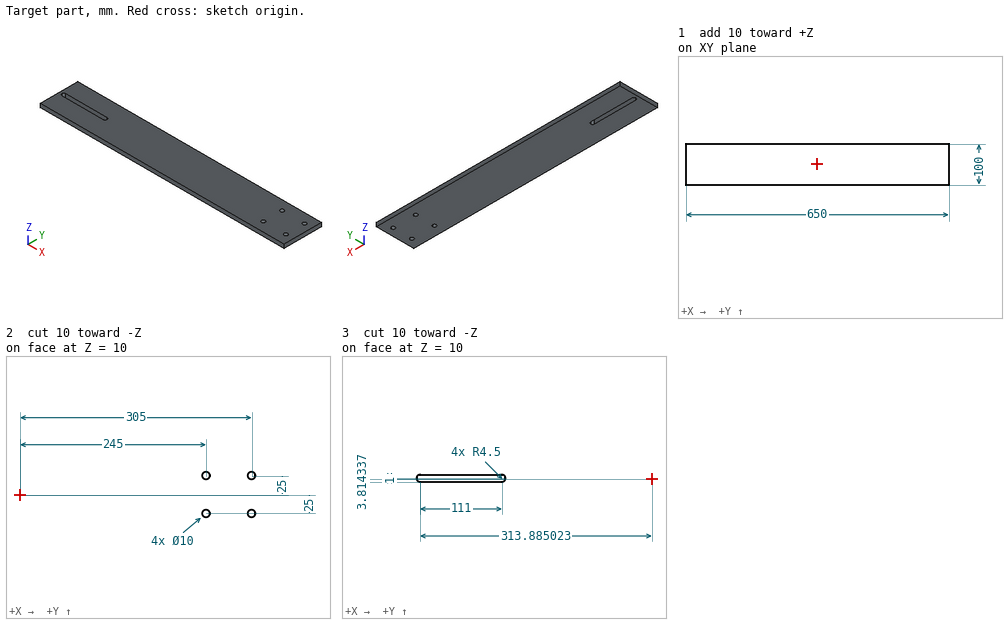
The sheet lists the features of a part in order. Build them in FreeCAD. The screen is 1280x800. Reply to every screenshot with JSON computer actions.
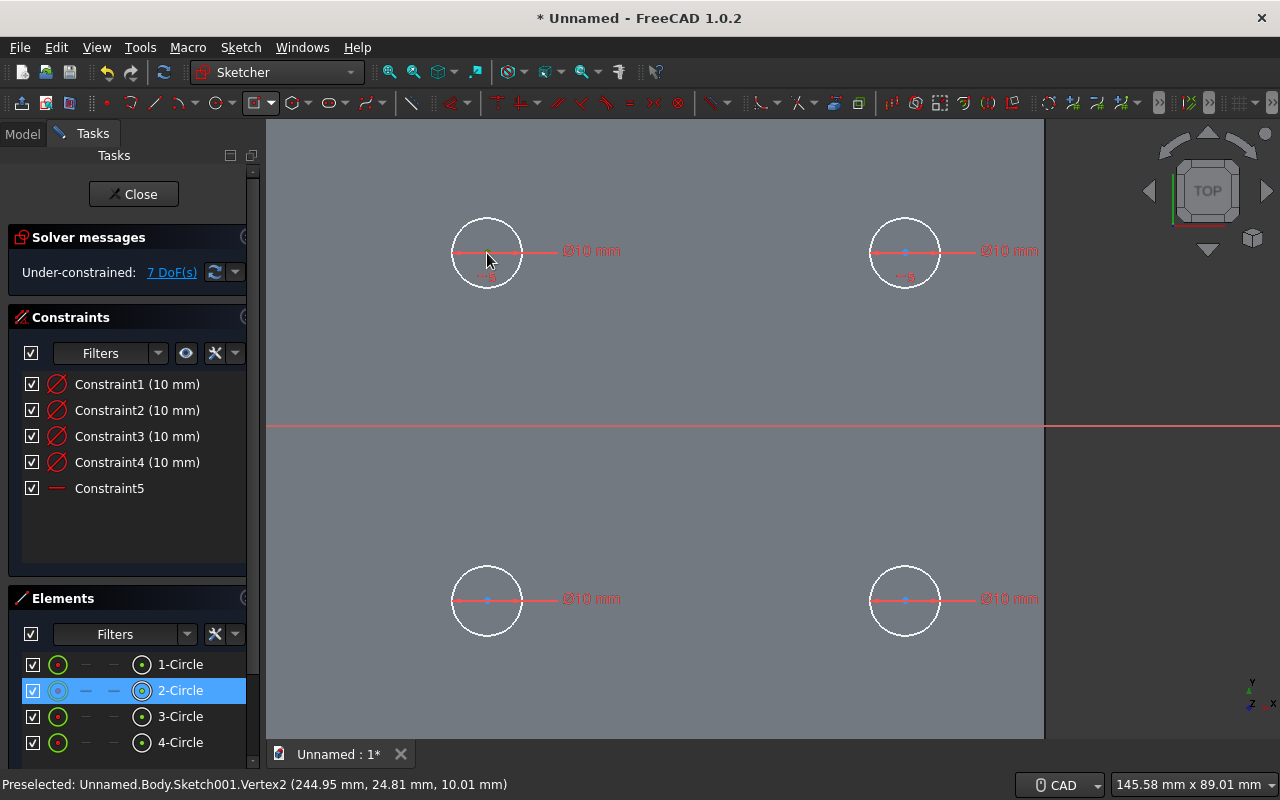
{"action": "left_click", "coordinate": [487, 601]}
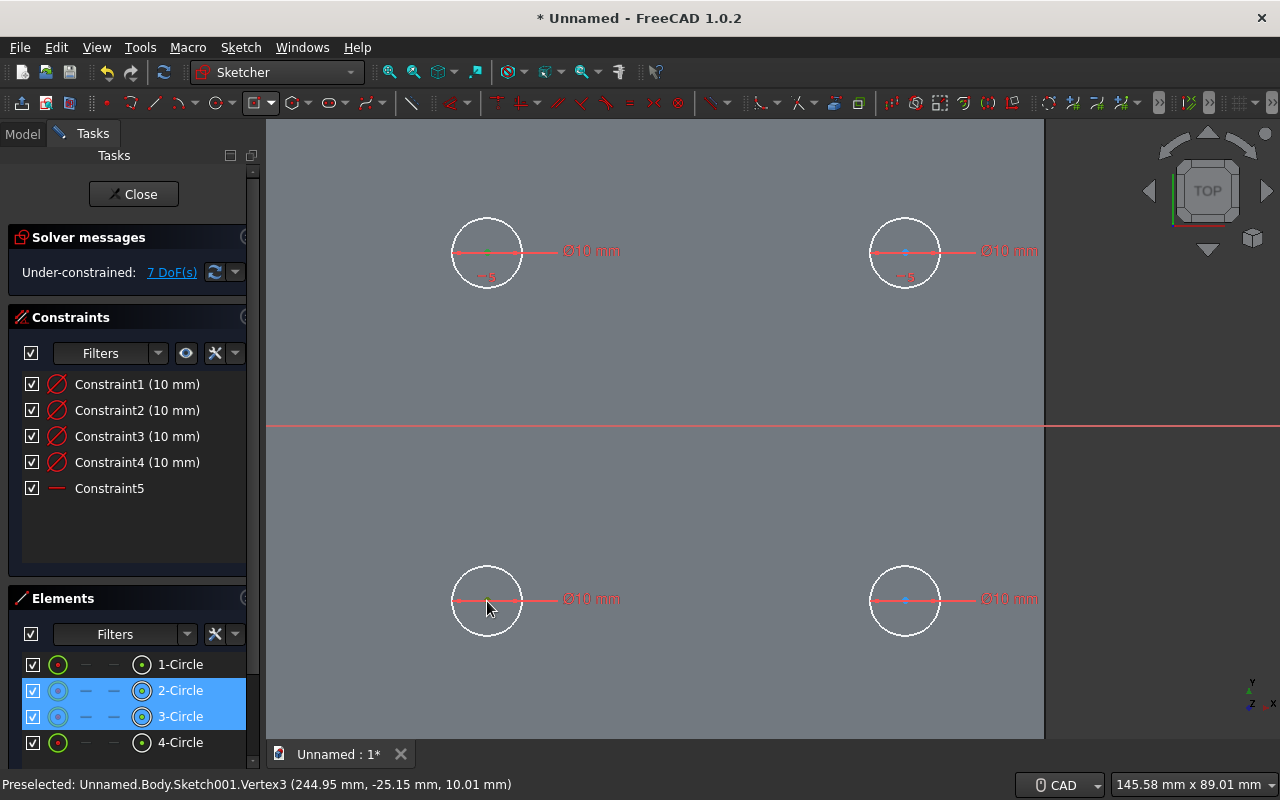
{"action": "key", "text": "v"}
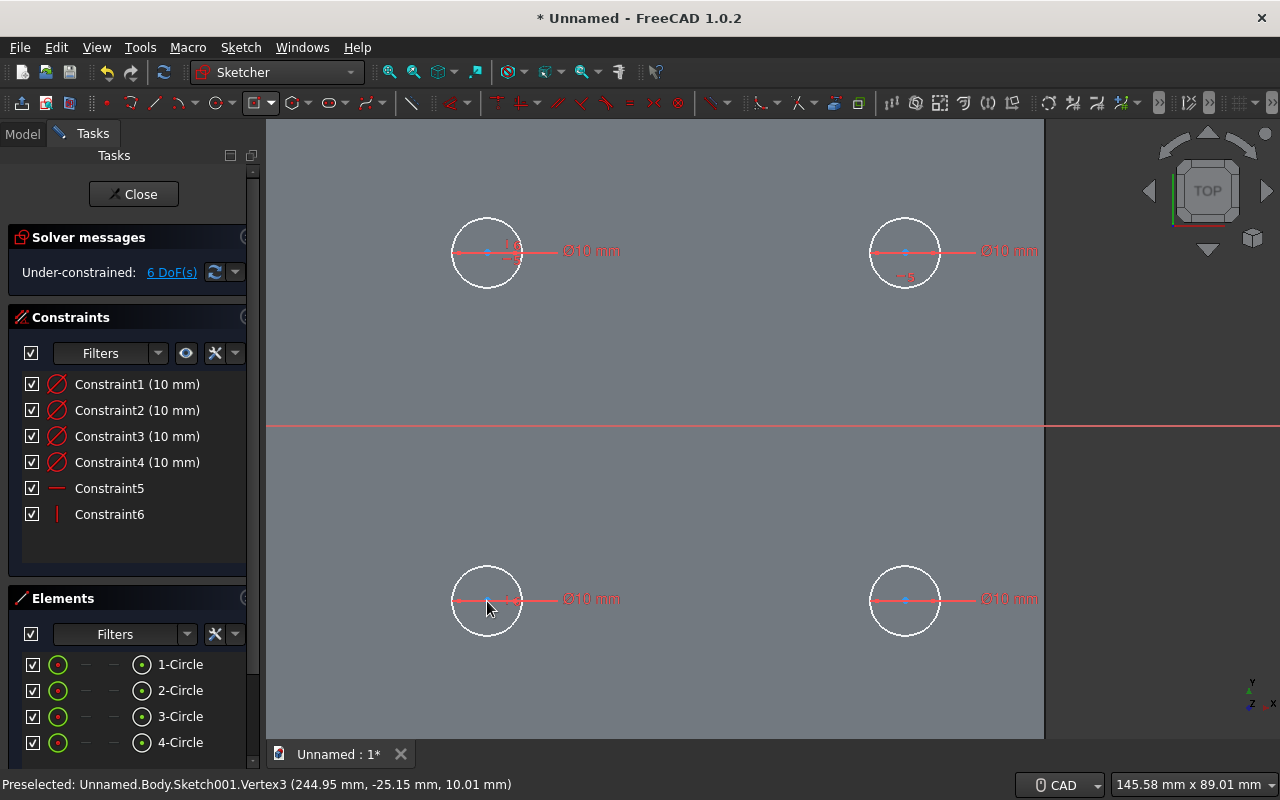
{"action": "left_click", "coordinate": [905, 253]}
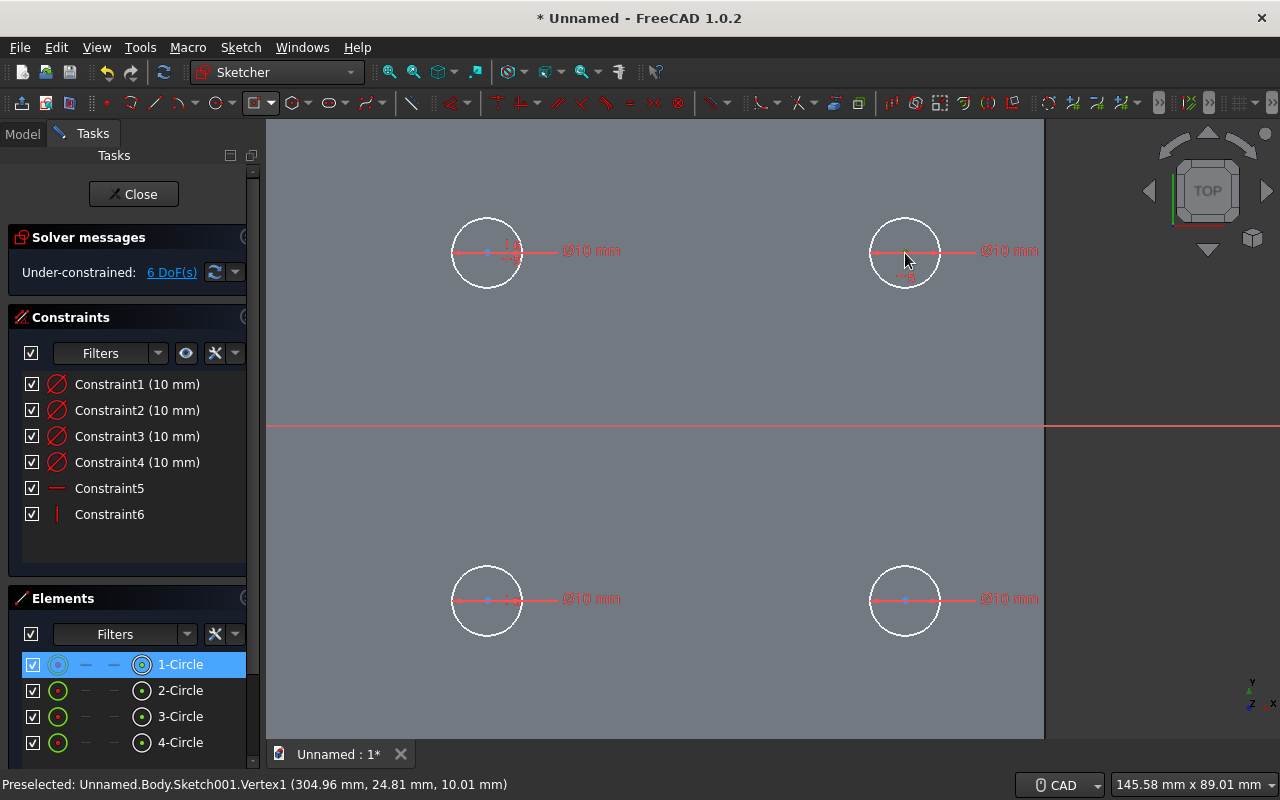
{"action": "left_click", "coordinate": [905, 601]}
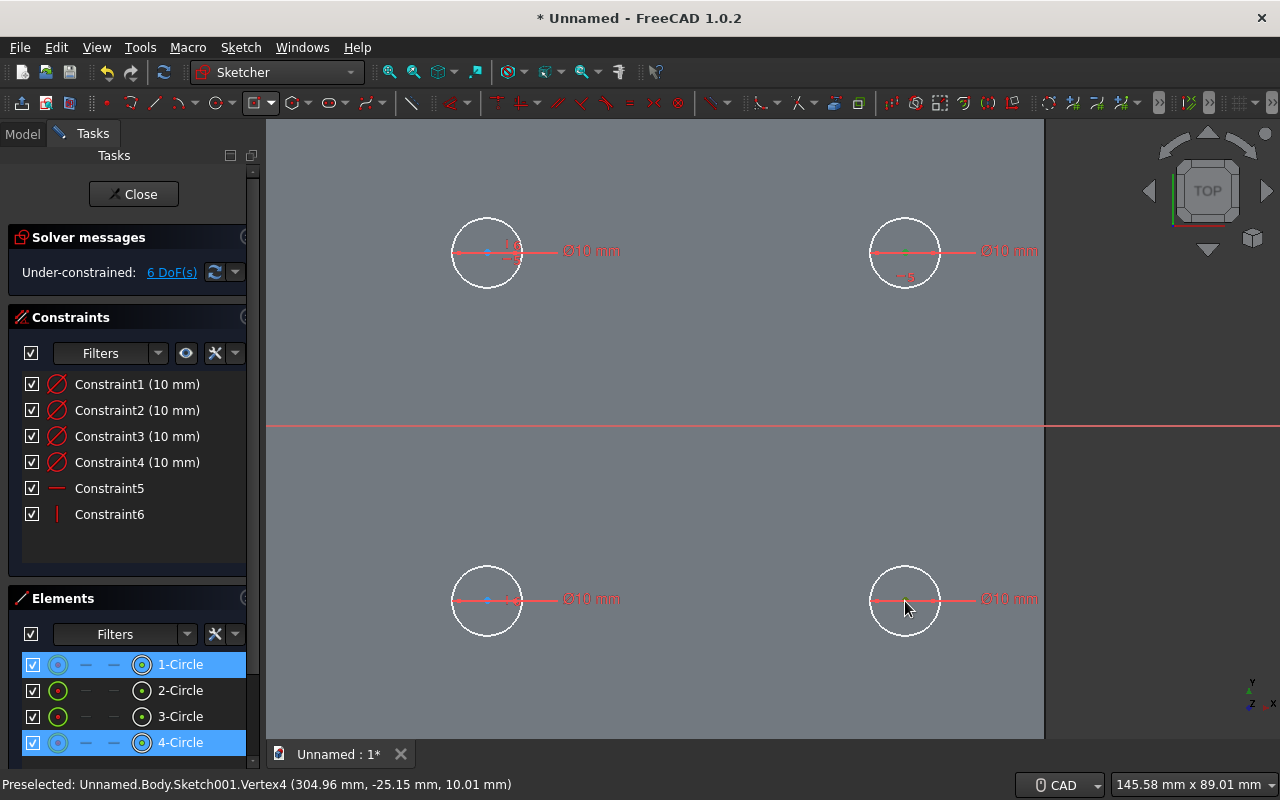
{"action": "key", "text": "v"}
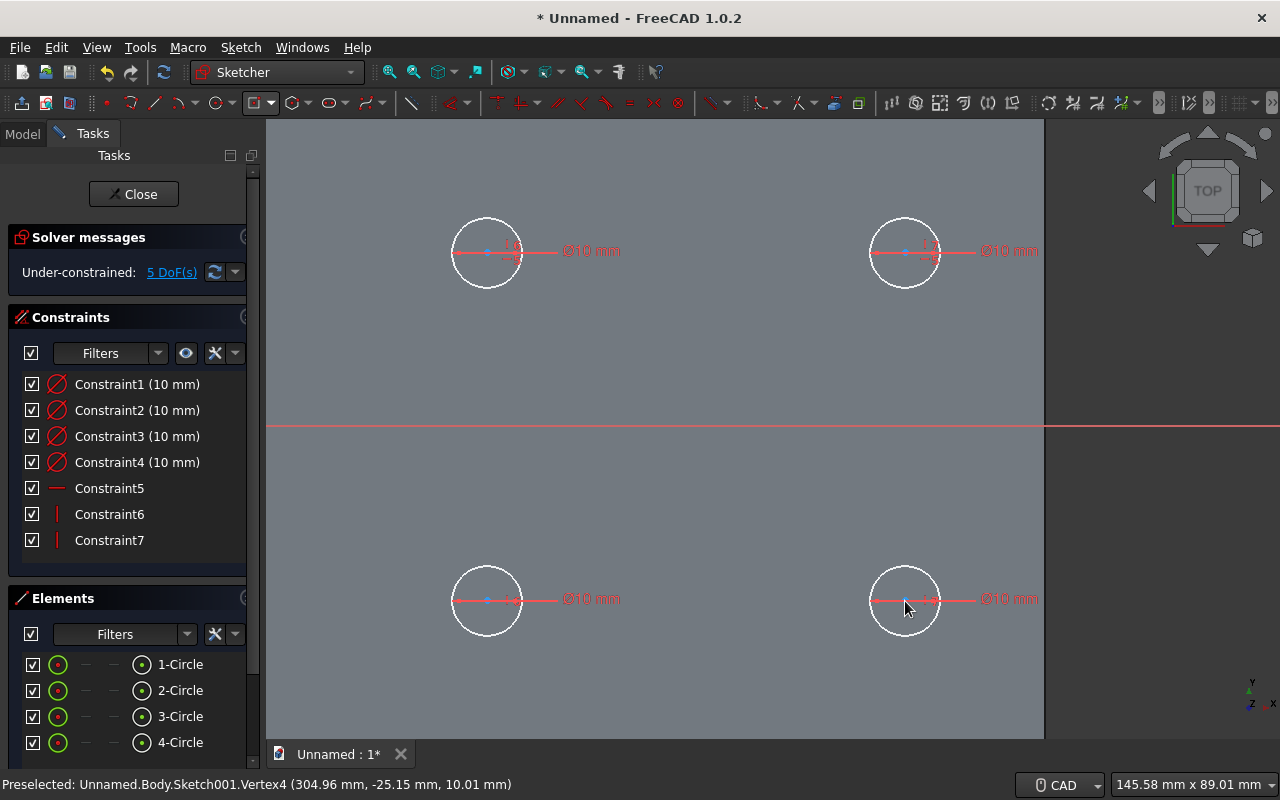
{"action": "left_click", "coordinate": [487, 601]}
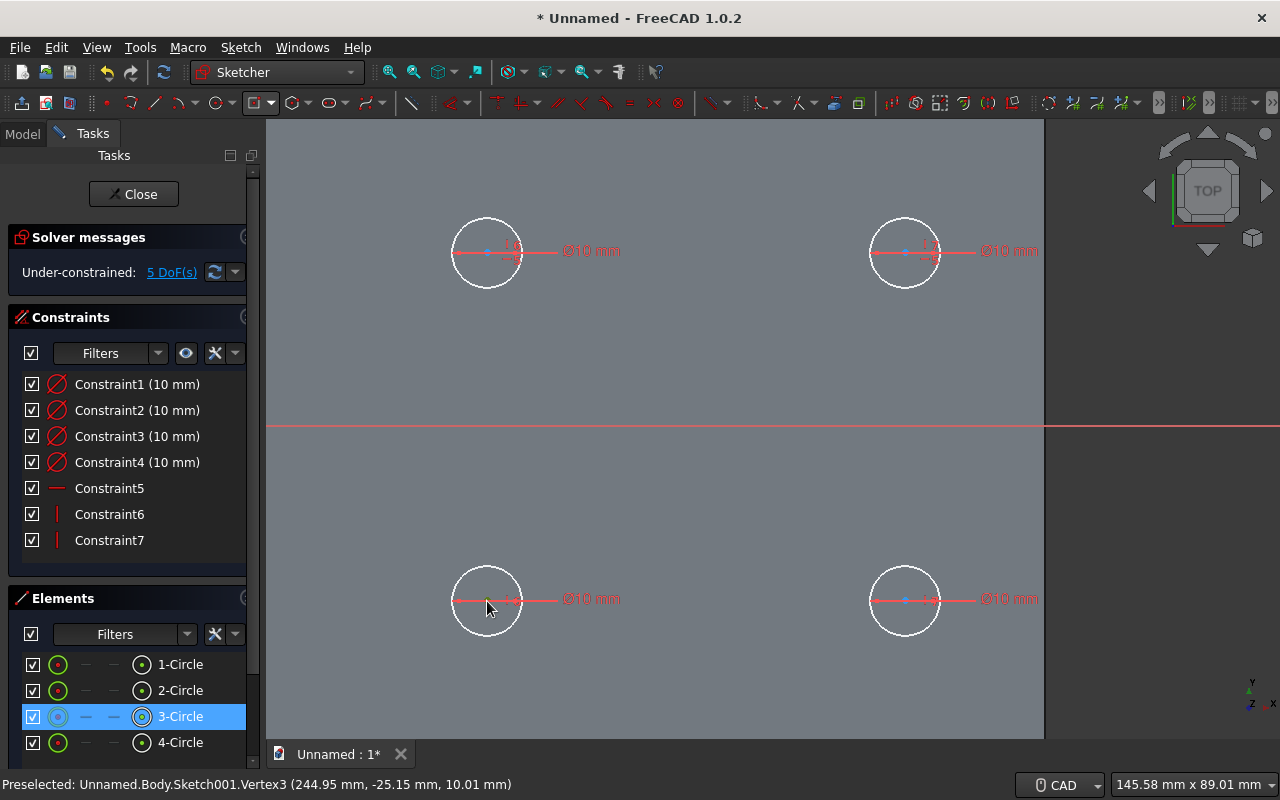
{"action": "left_click", "coordinate": [905, 601]}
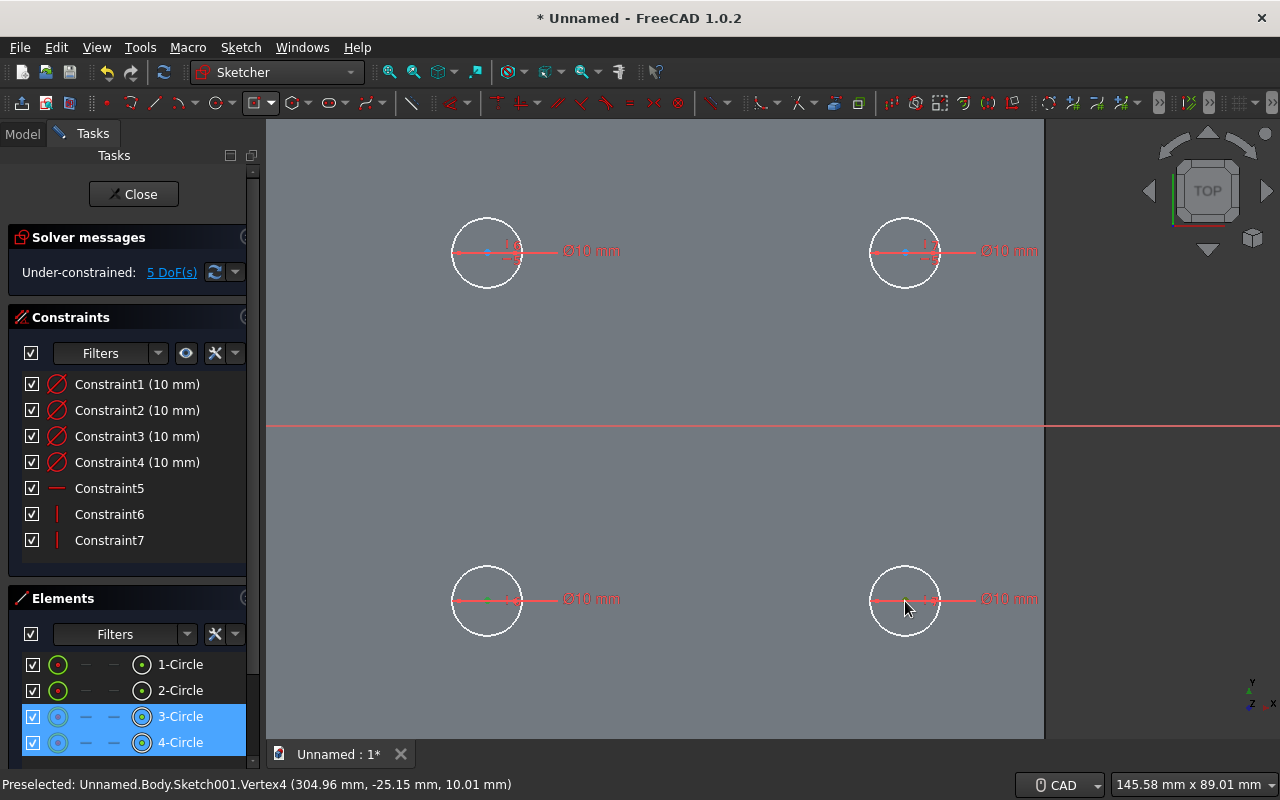
{"action": "key", "text": "h"}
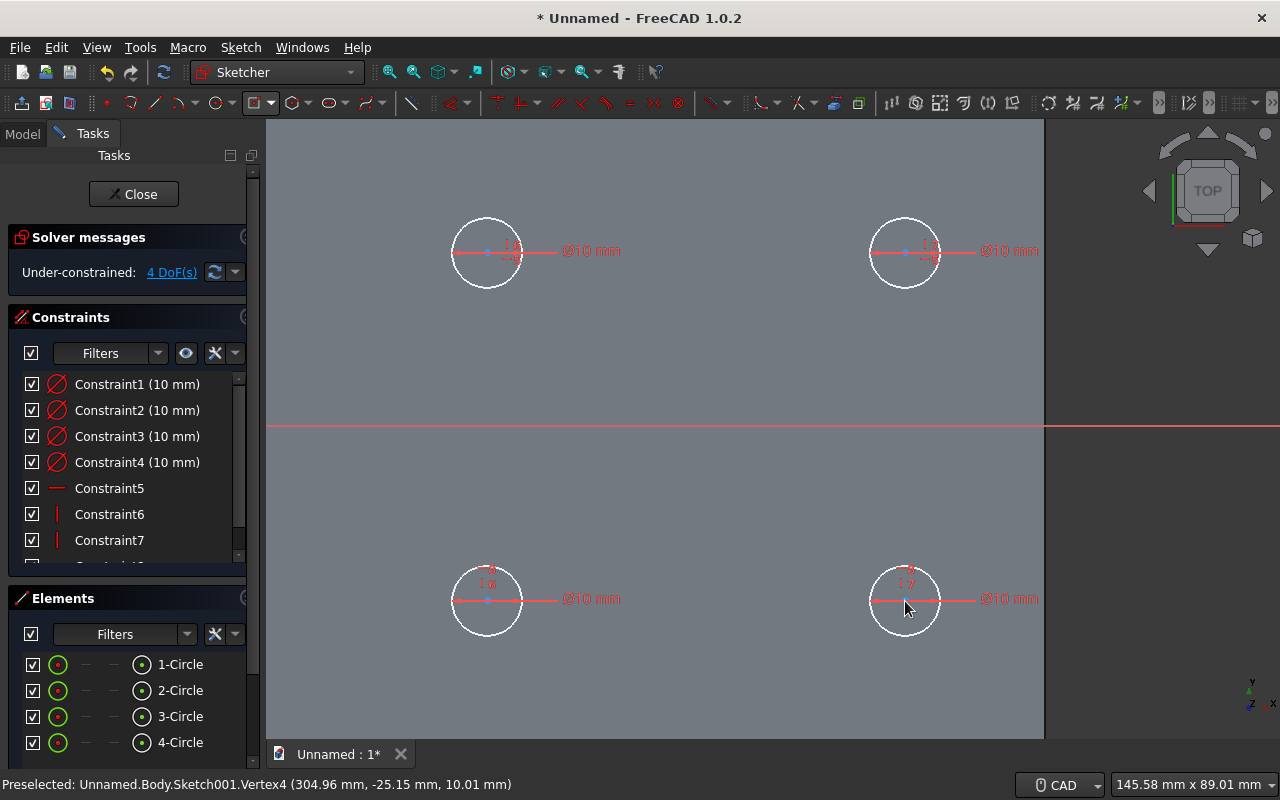
{"action": "key", "text": "d"}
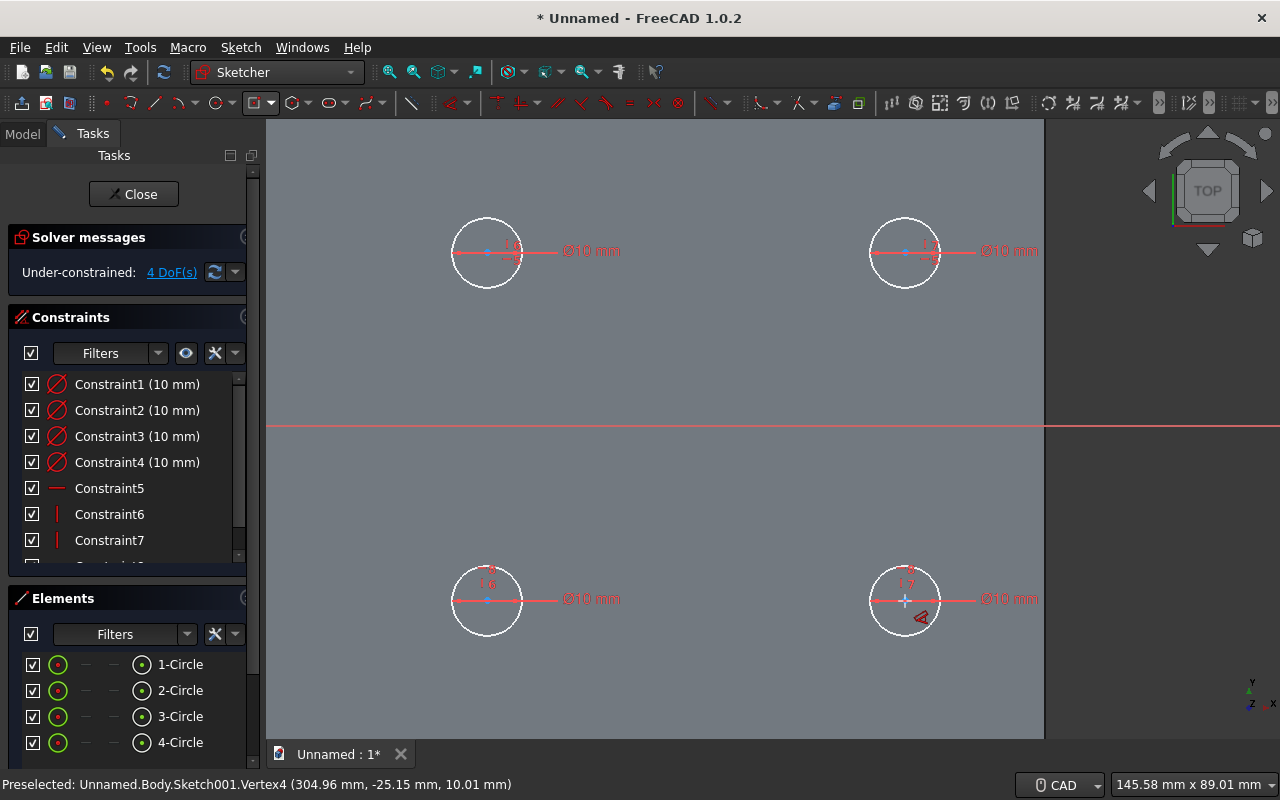
{"action": "left_click", "coordinate": [905, 253]}
{"action": "left_click", "coordinate": [939, 339]}